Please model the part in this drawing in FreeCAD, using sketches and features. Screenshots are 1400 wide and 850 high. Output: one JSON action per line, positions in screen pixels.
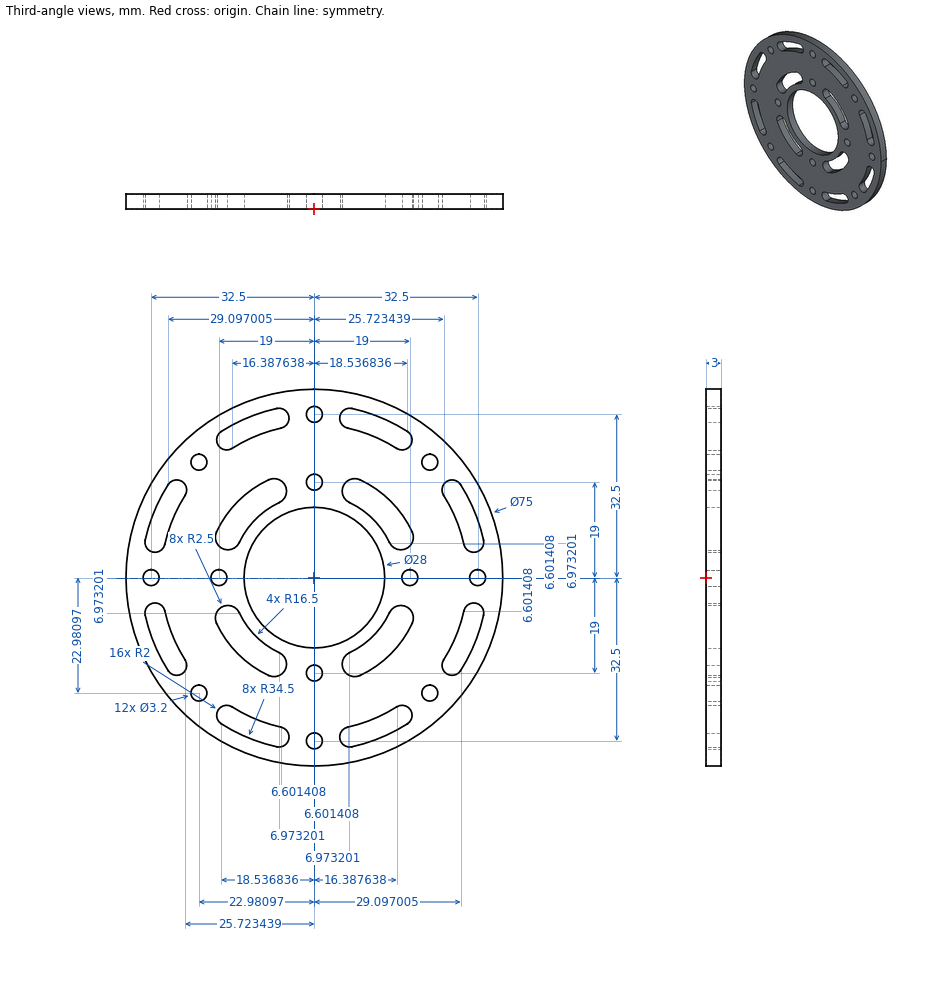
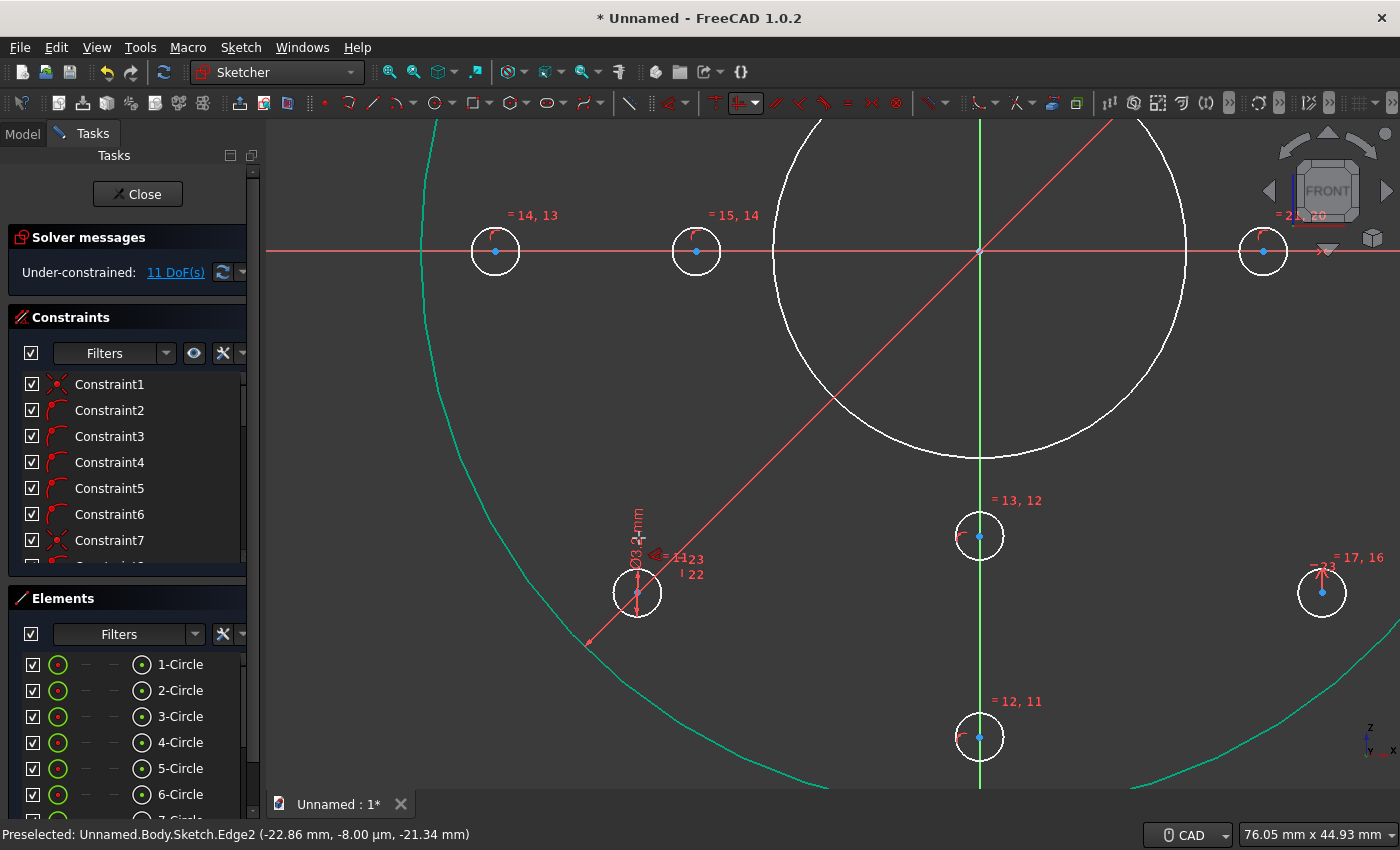
{"action": "left_click", "coordinate": [834, 398]}
{"action": "left_click", "coordinate": [811, 421]}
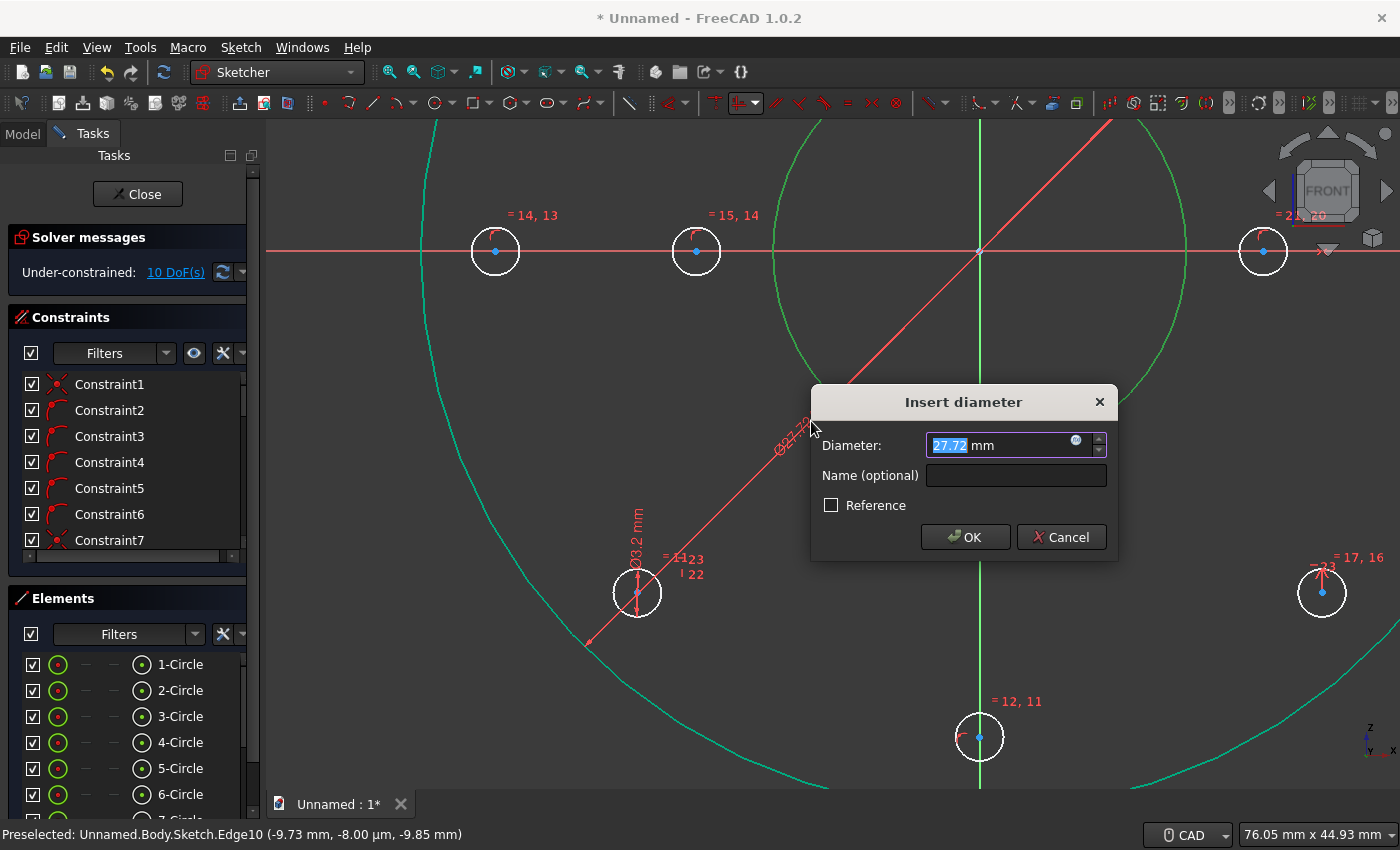
{"action": "type", "text": "28"}
{"action": "key", "text": "Return"}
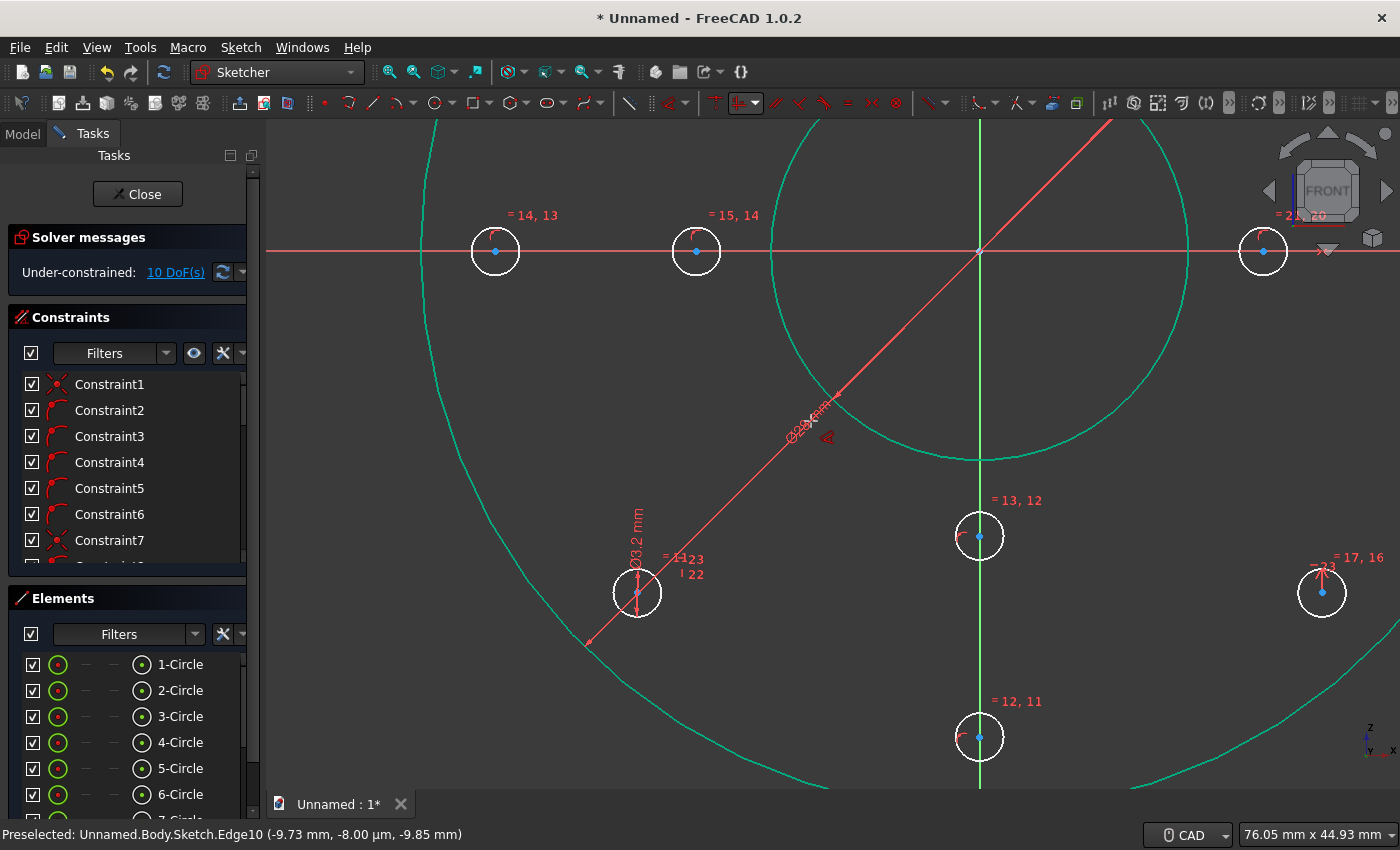
{"action": "left_click", "coordinate": [980, 536]}
{"action": "left_click", "coordinate": [1014, 394]}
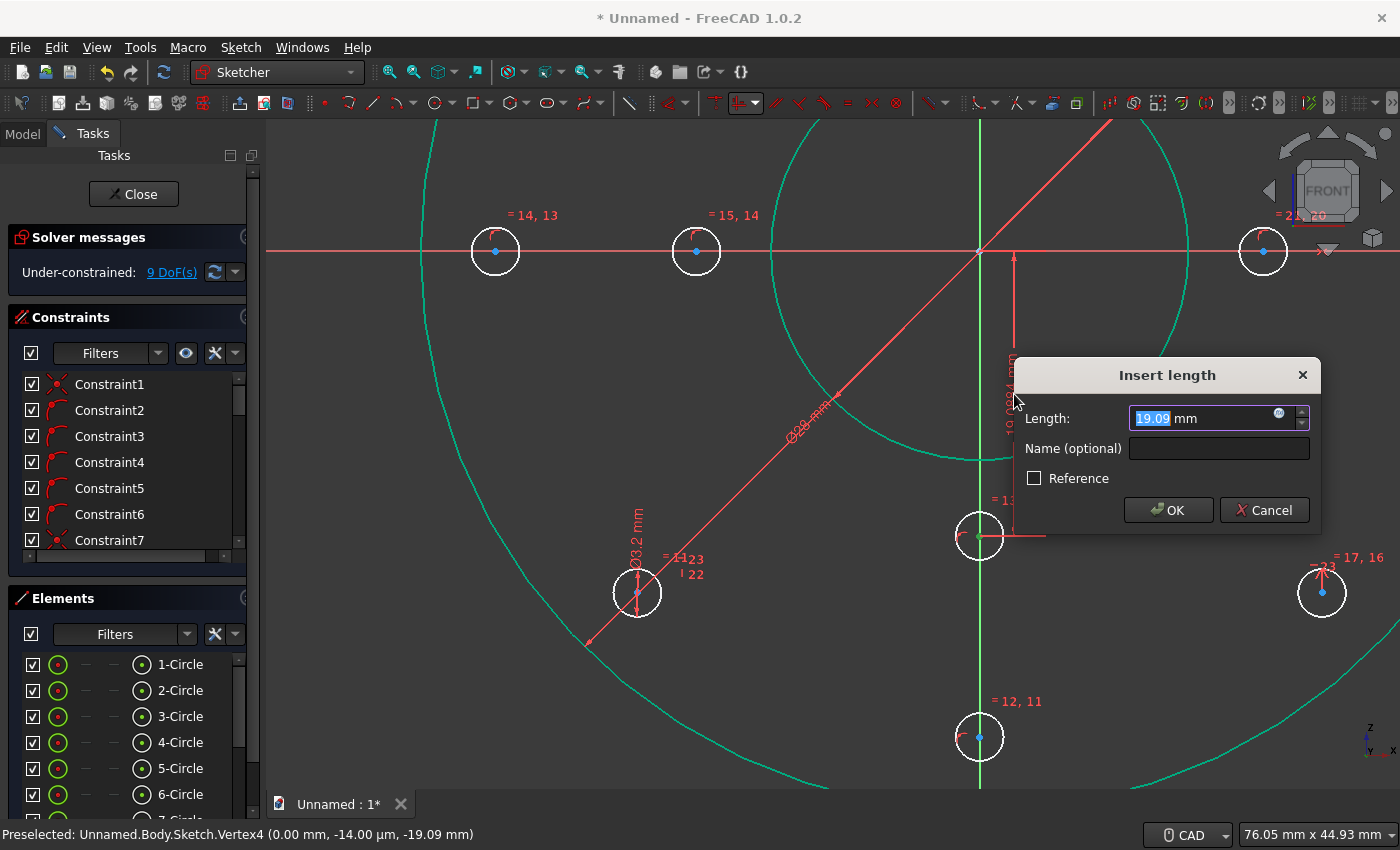
{"action": "type", "text": "19"}
{"action": "key", "text": "Return"}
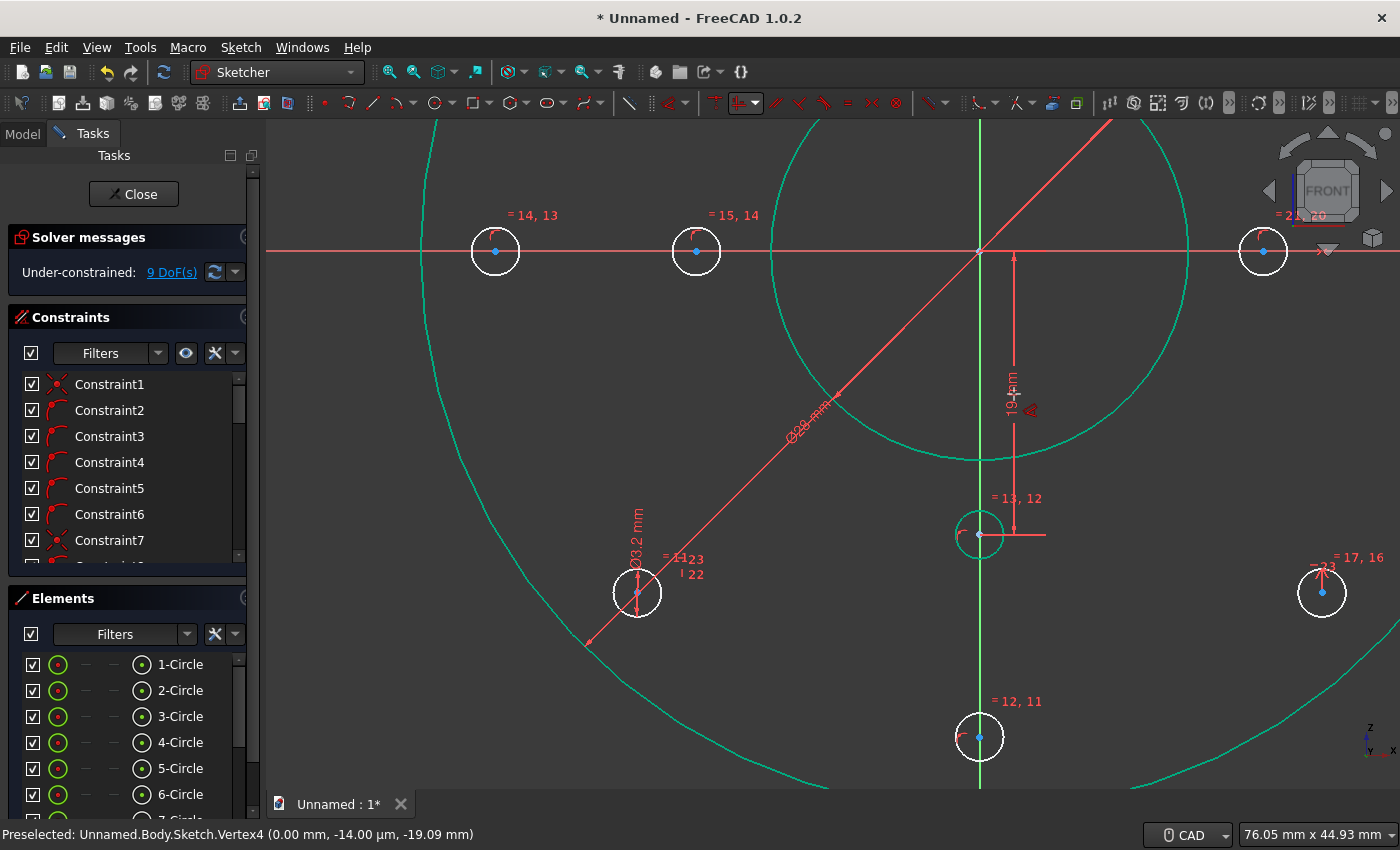
{"action": "left_click", "coordinate": [696, 251]}
{"action": "left_click", "coordinate": [838, 285]}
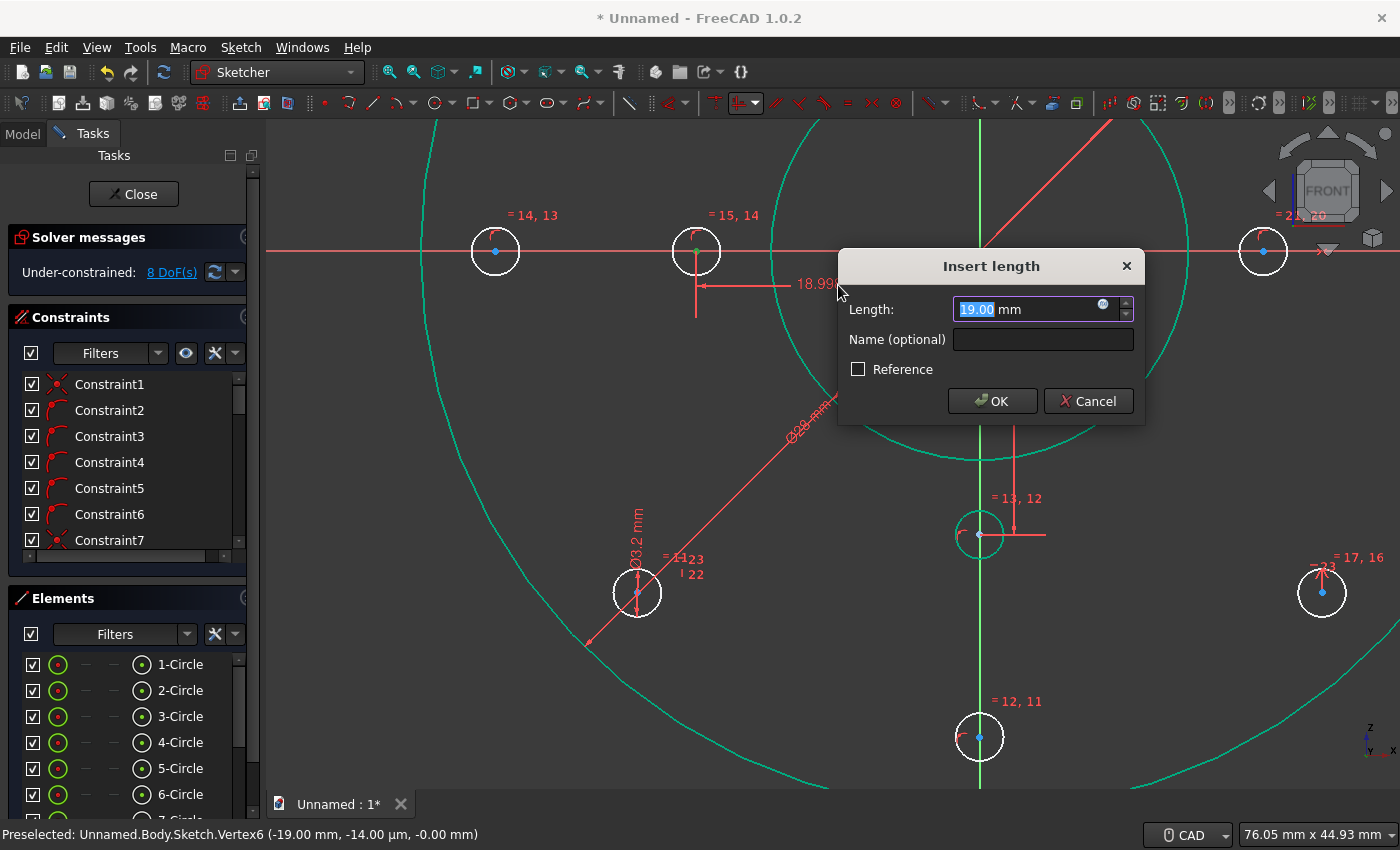
{"action": "type", "text": "19"}
{"action": "key", "text": "Return"}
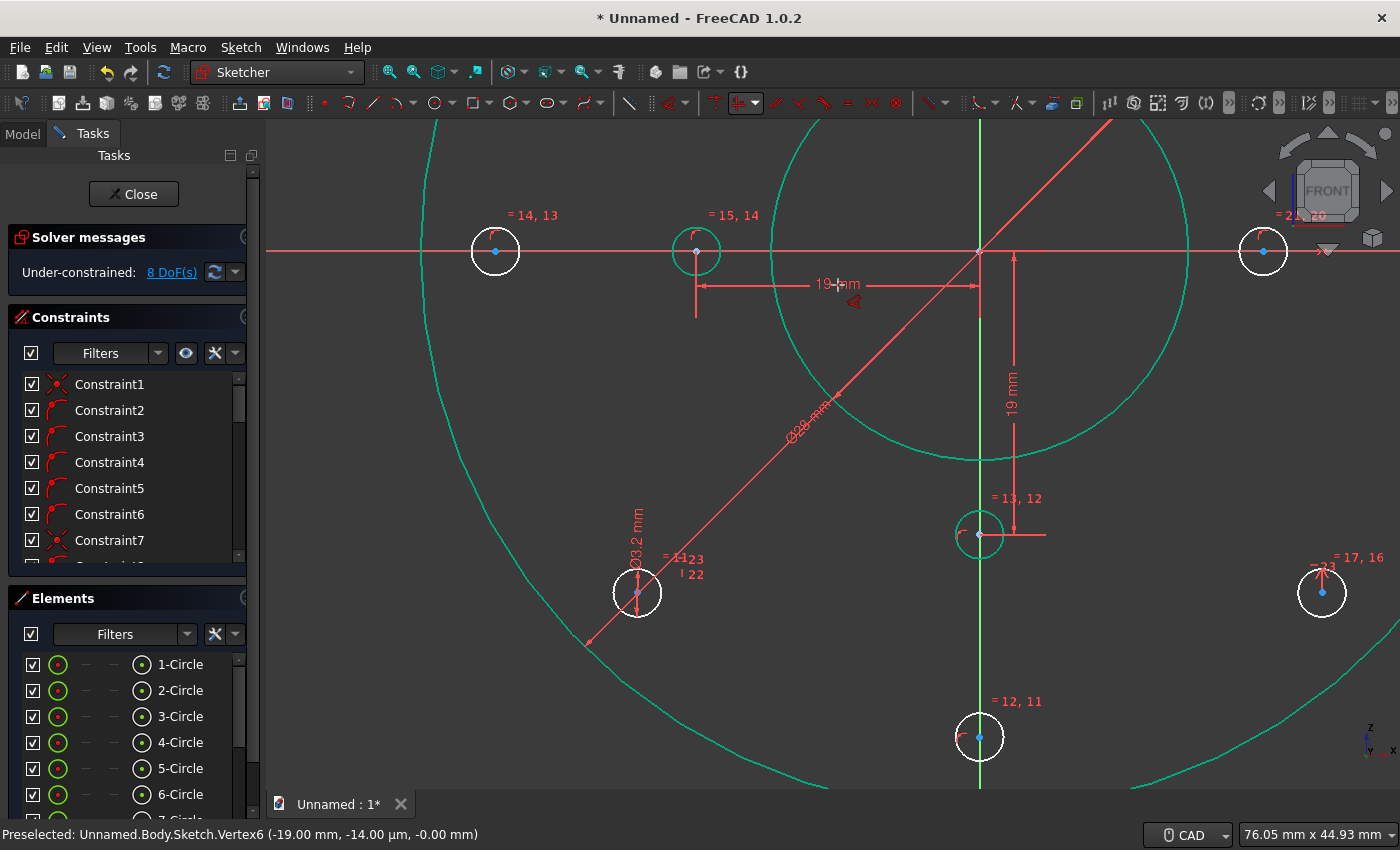
{"action": "scroll", "coordinate": [639, 572], "scroll_direction": "down", "scroll_amount": 5}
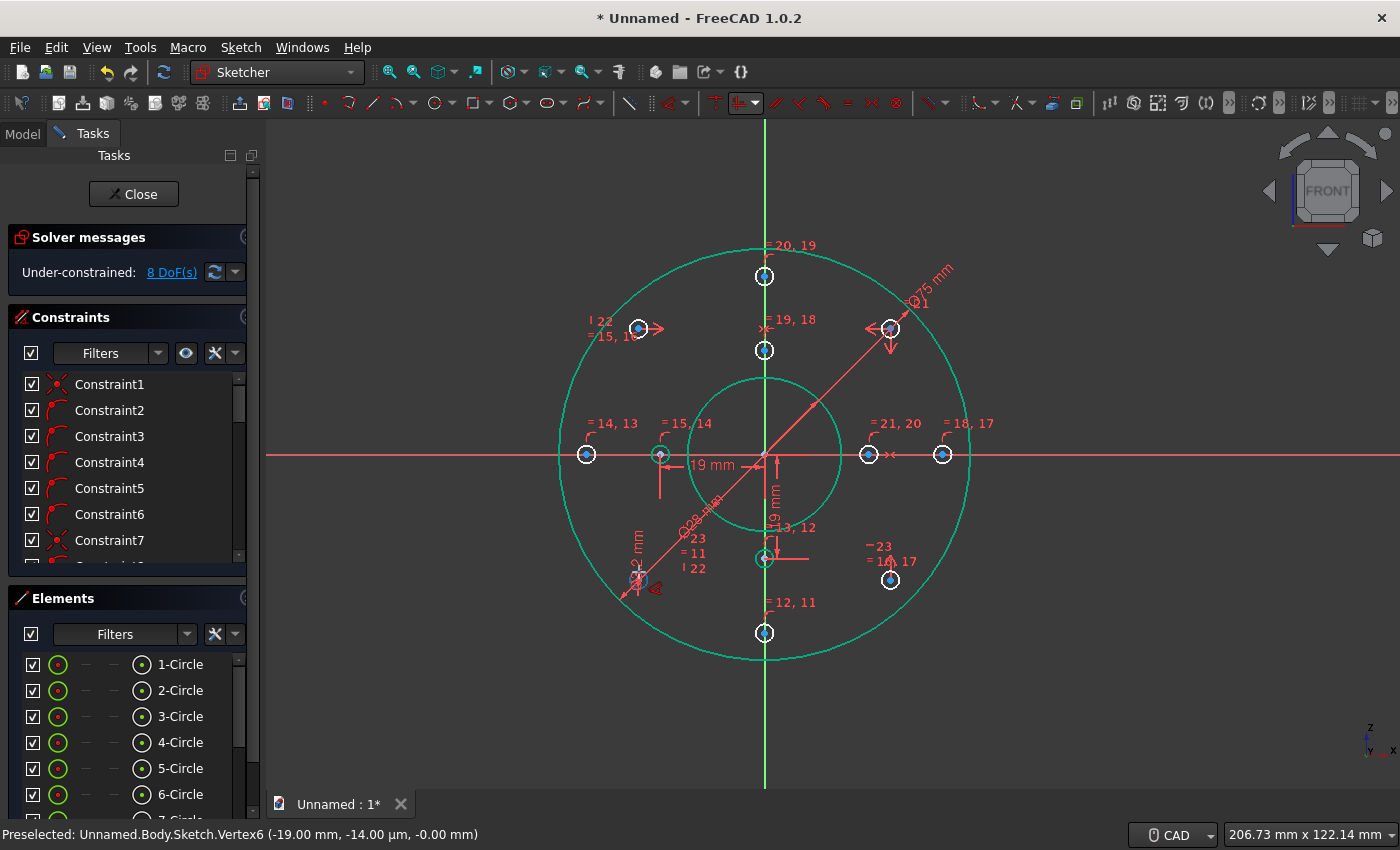
{"action": "left_click", "coordinate": [765, 351]}
{"action": "left_click", "coordinate": [799, 403]}